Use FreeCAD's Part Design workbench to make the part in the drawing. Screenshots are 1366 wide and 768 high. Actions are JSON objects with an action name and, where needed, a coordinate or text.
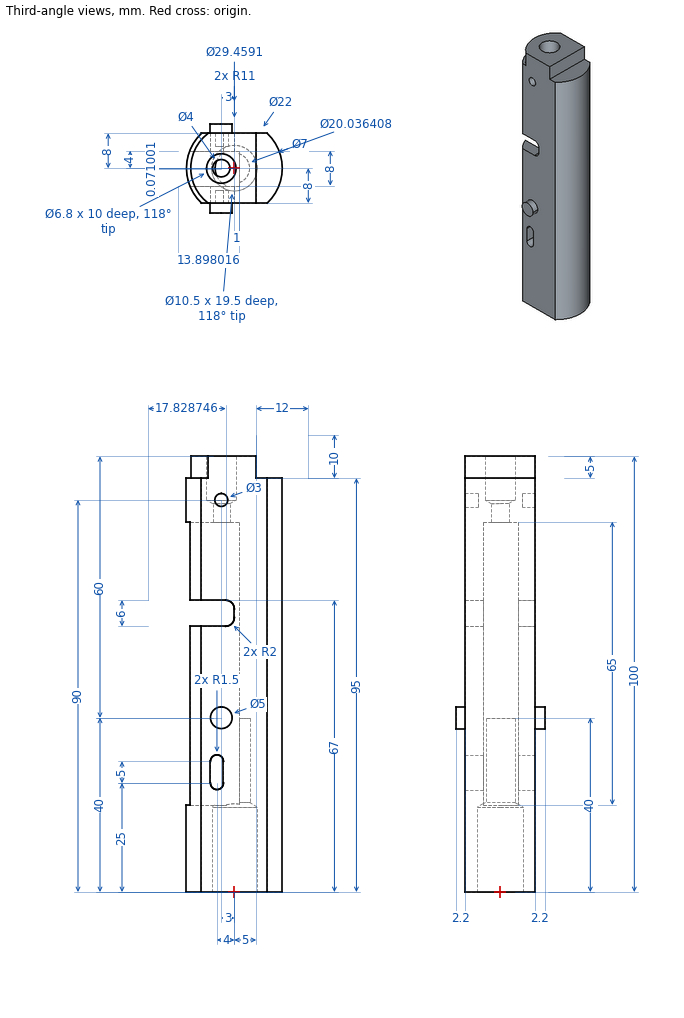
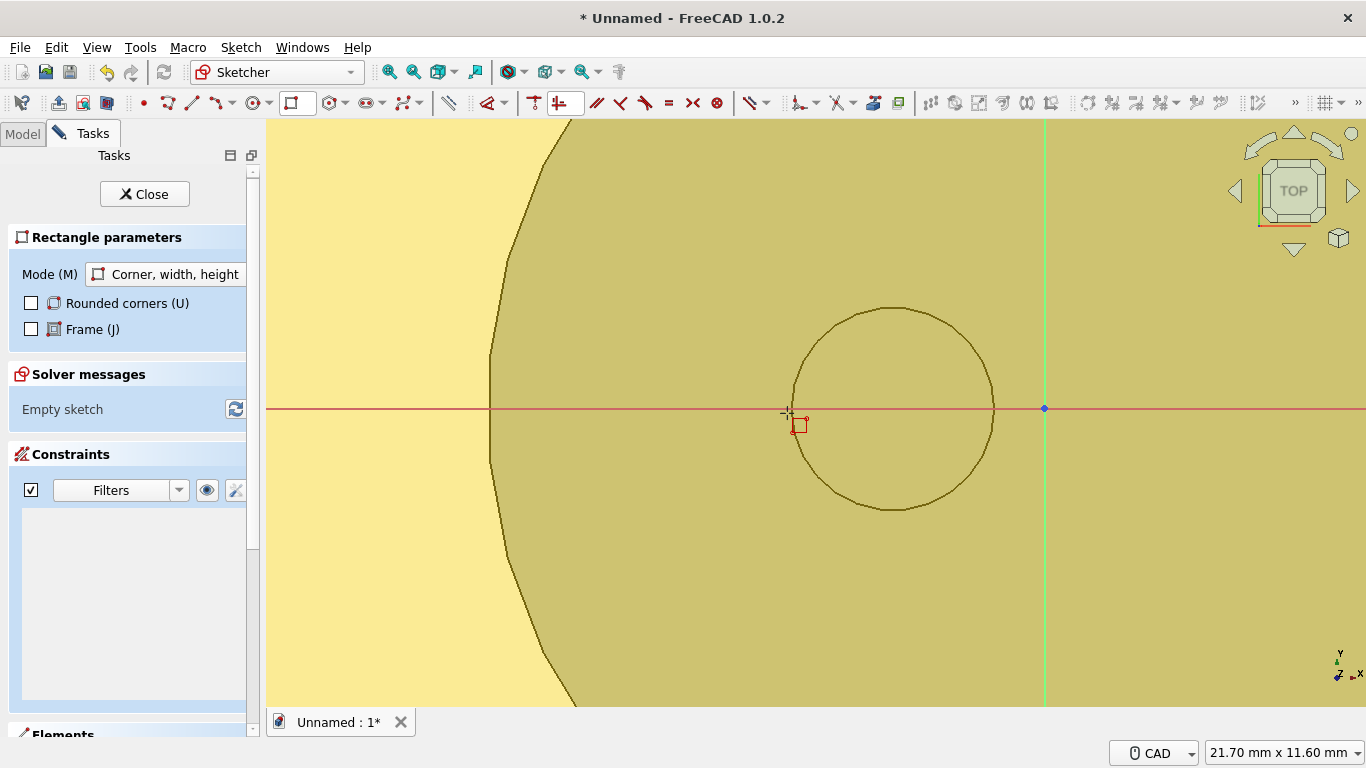
{"action": "left_click", "coordinate": [391, 206]}
{"action": "mouse_move", "coordinate": [1096, 612]}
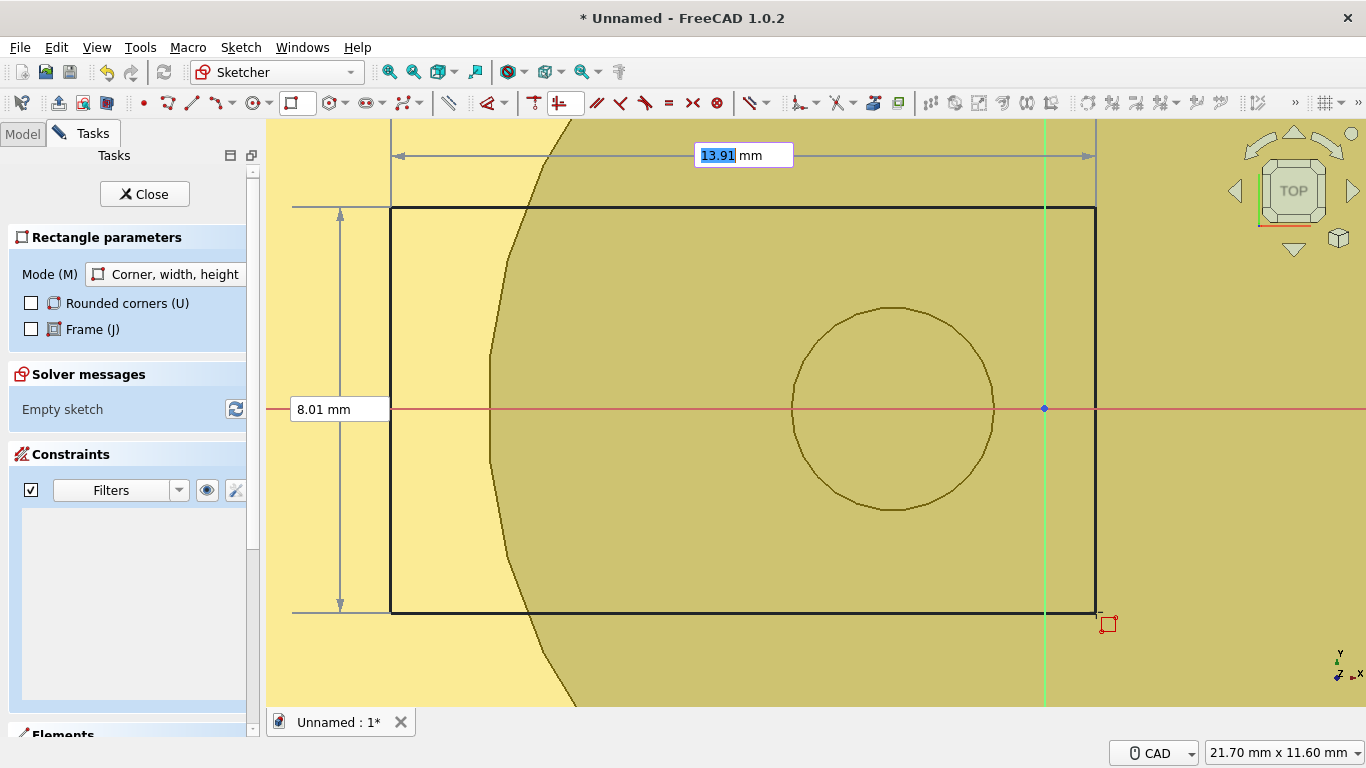
{"action": "type", "text": "13.898016"}
{"action": "key", "text": "Tab"}
{"action": "type", "text": "8"}
{"action": "key", "text": "Return"}
{"action": "key", "text": "Escape"}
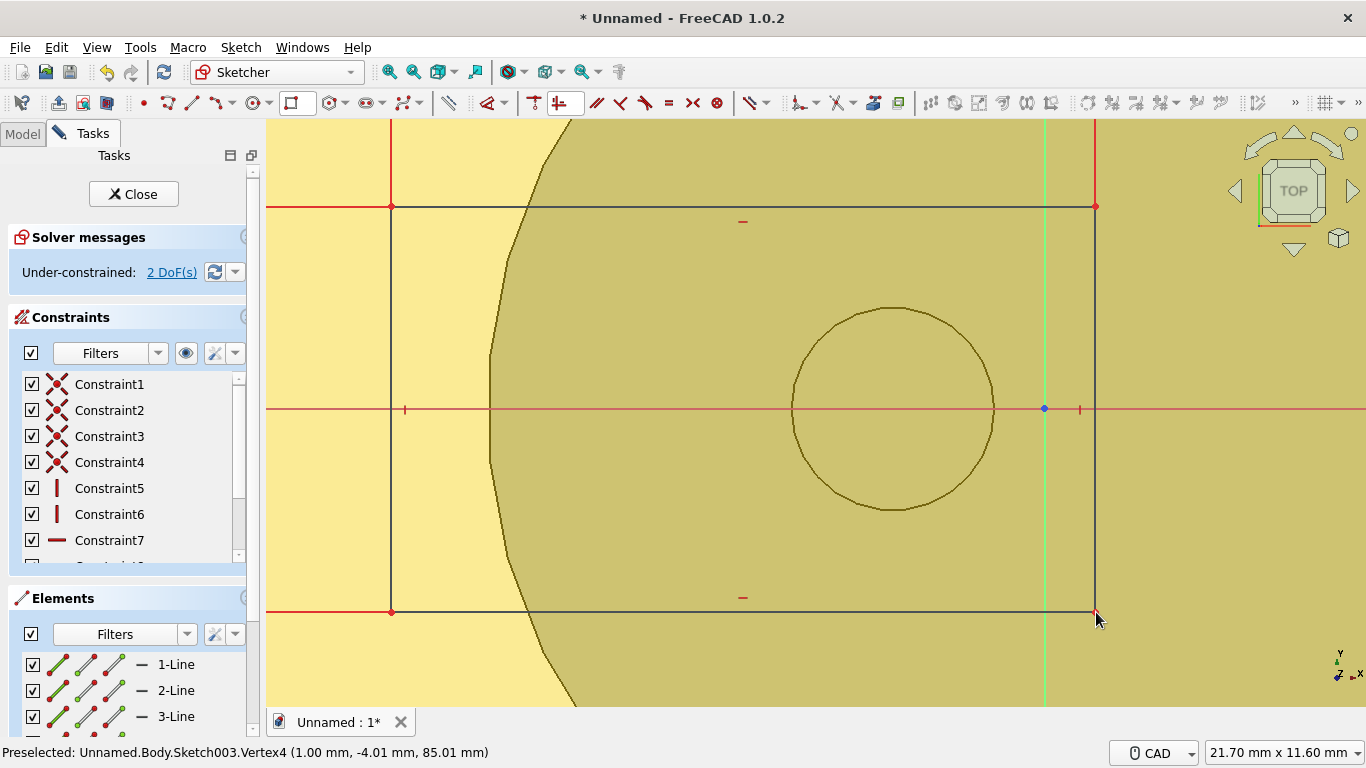
{"action": "key", "text": "d"}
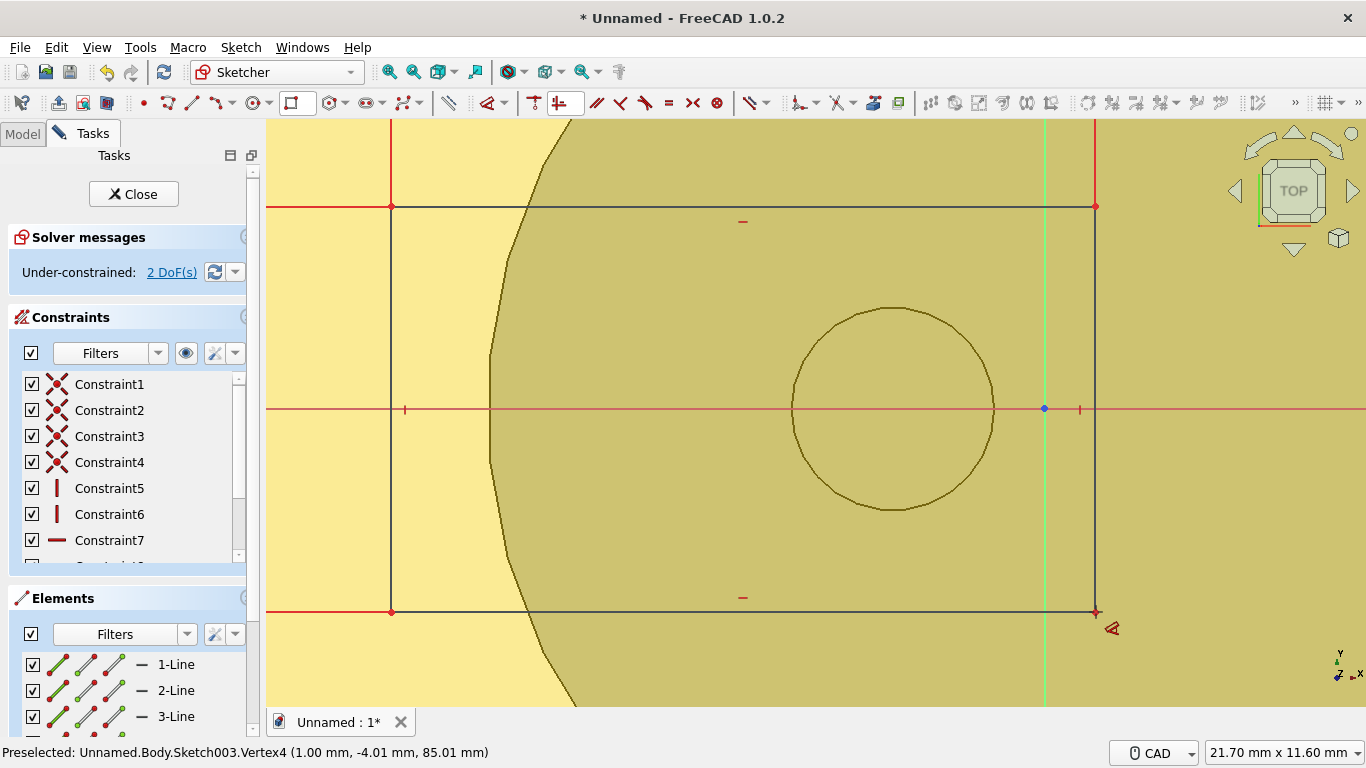
{"action": "left_click", "coordinate": [391, 207]}
{"action": "left_click", "coordinate": [357, 308]}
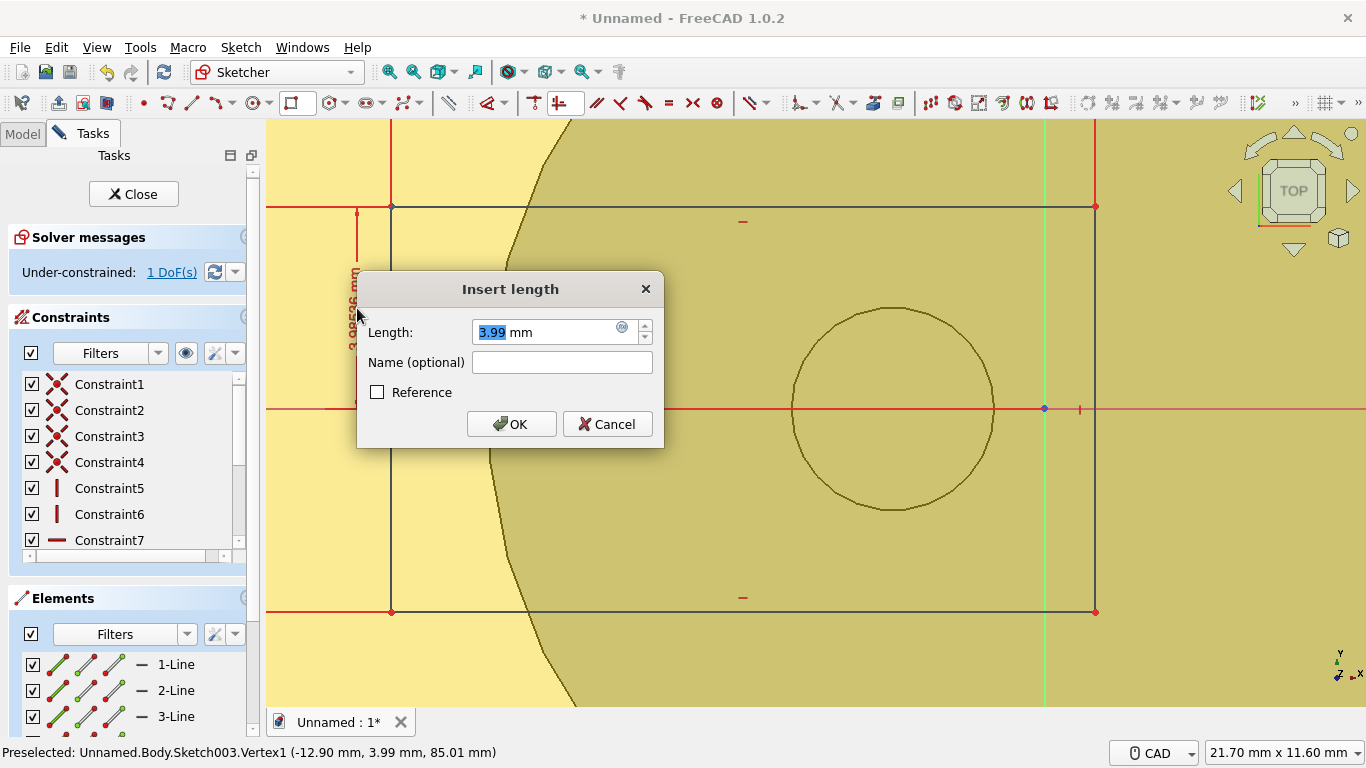
{"action": "type", "text": "4"}
{"action": "key", "text": "Return"}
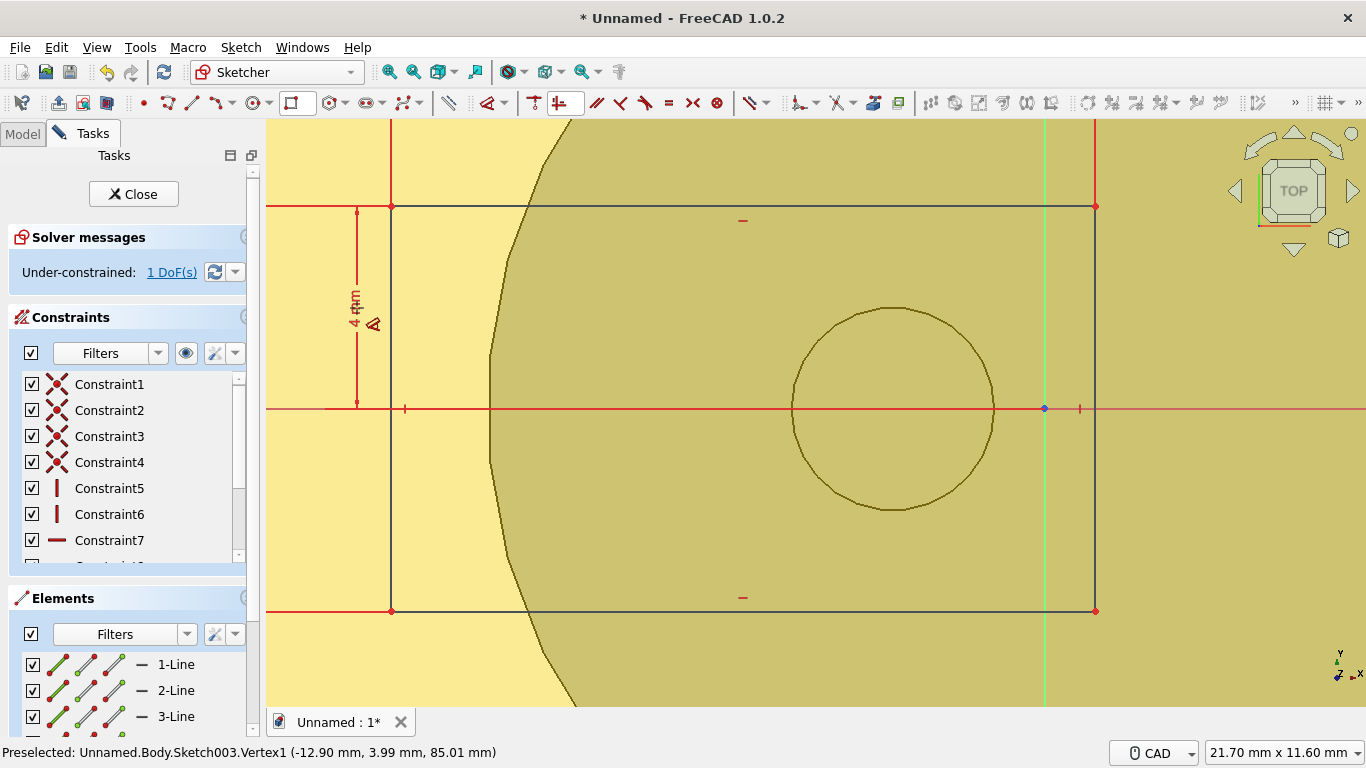
{"action": "left_click", "coordinate": [1095, 612]}
{"action": "left_click", "coordinate": [1070, 646]}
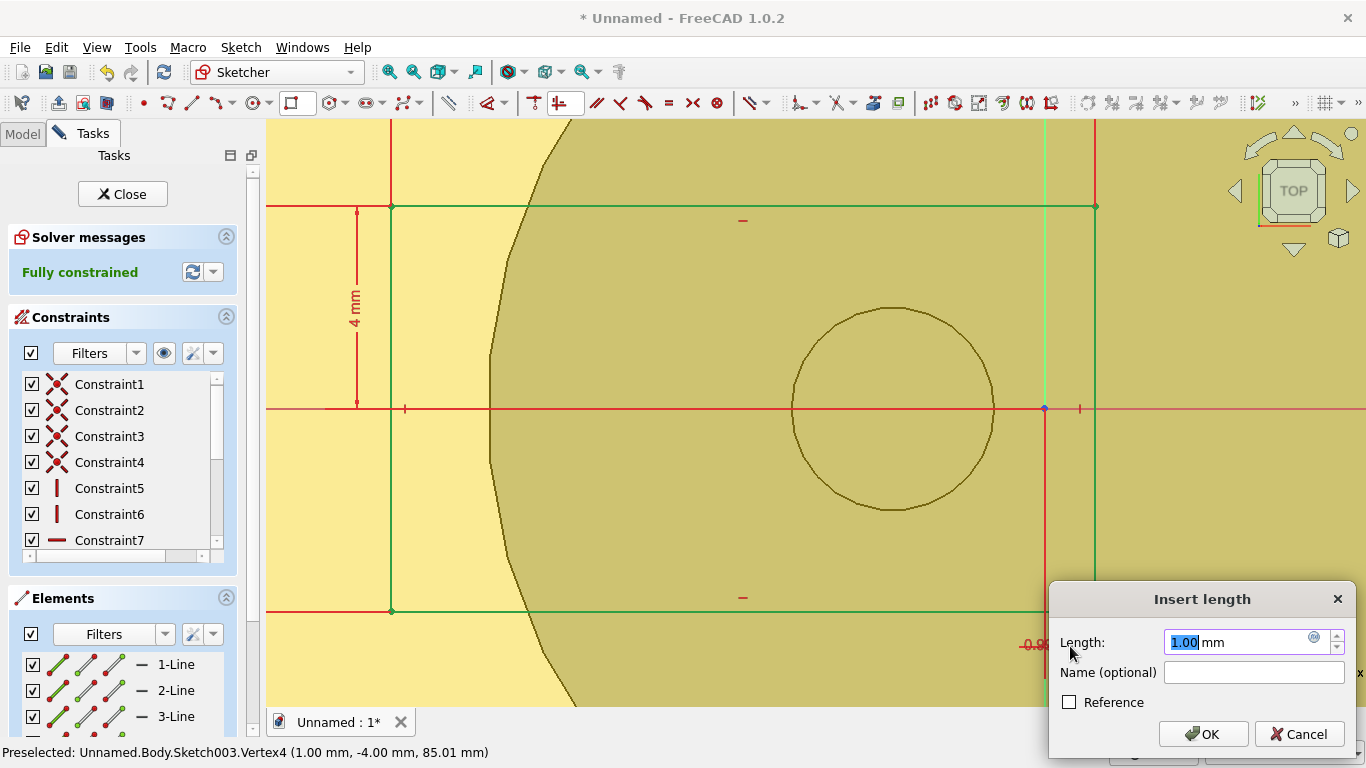
{"action": "type", "text": "1"}
{"action": "key", "text": "Return"}
{"action": "key", "text": "Escape"}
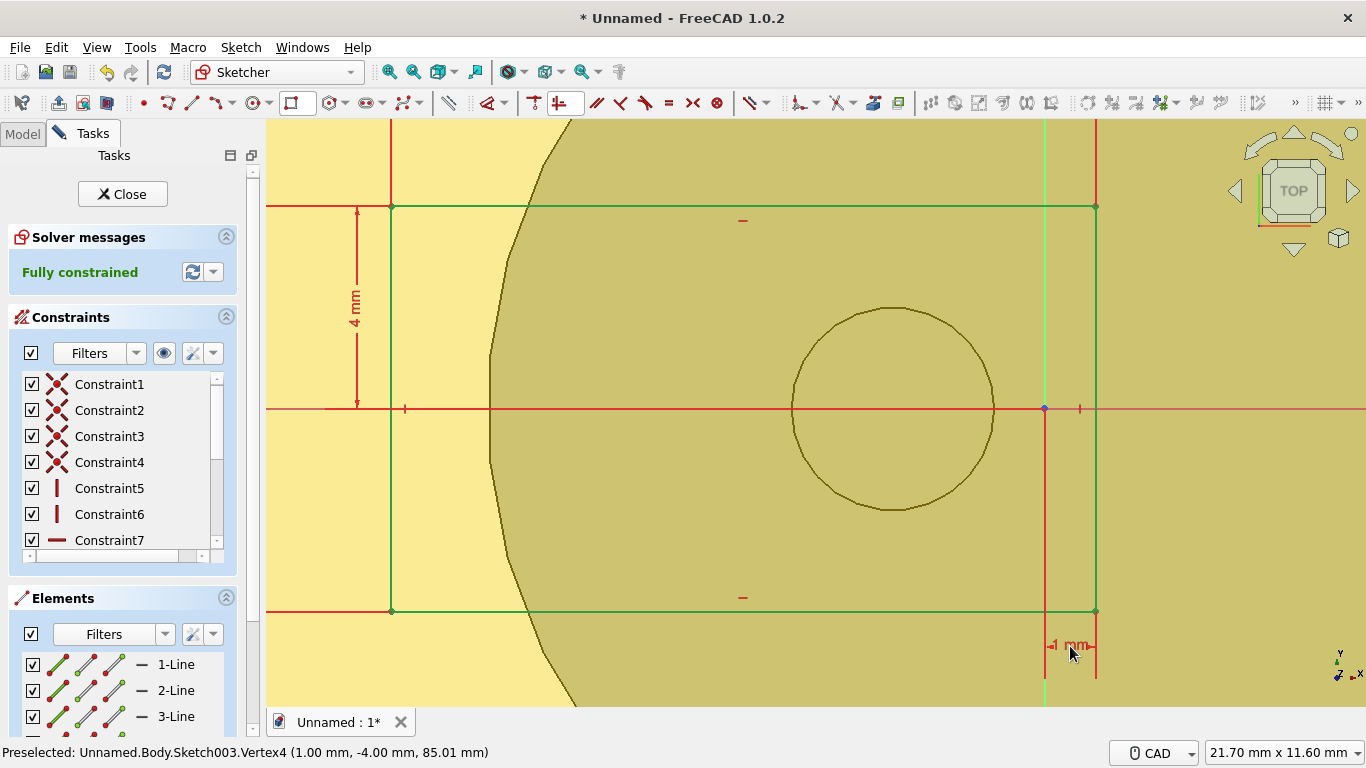
{"action": "left_click", "coordinate": [123, 194]}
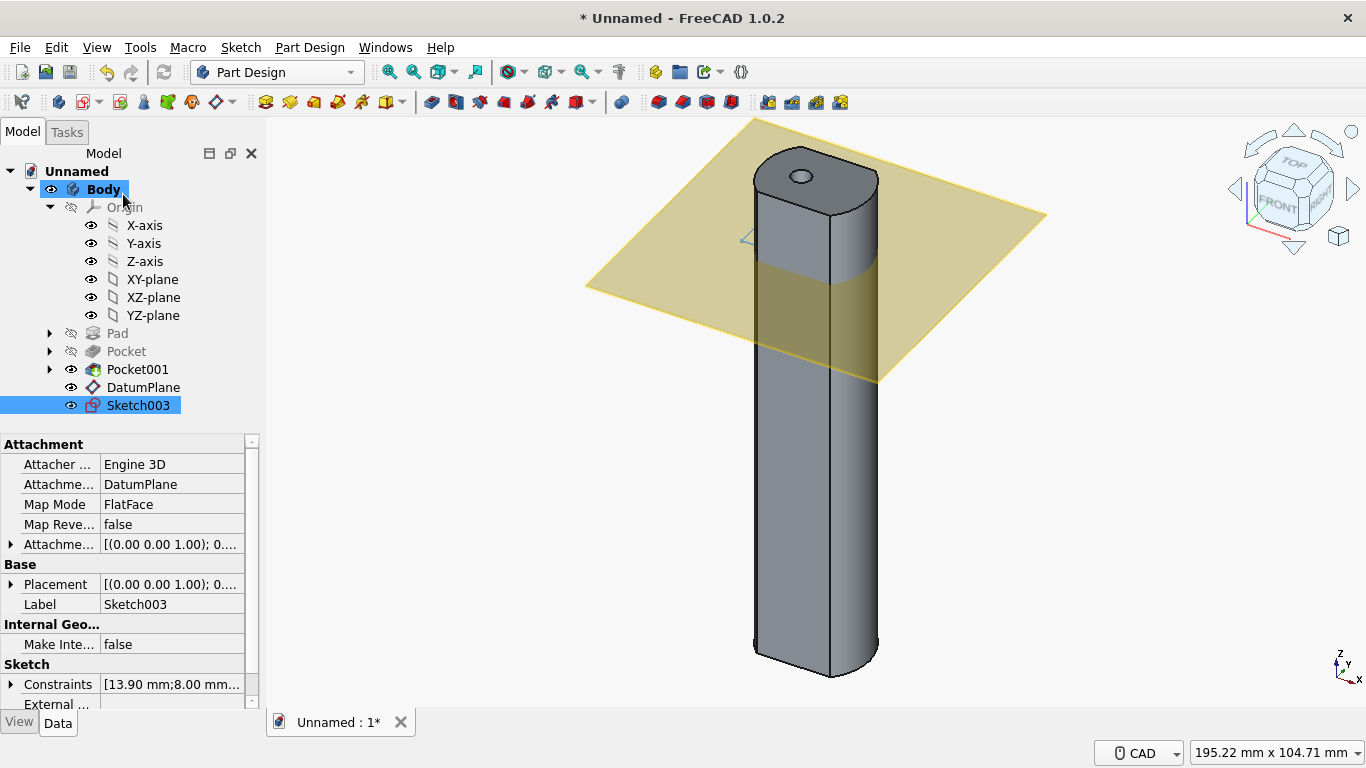
{"action": "left_click", "coordinate": [432, 102]}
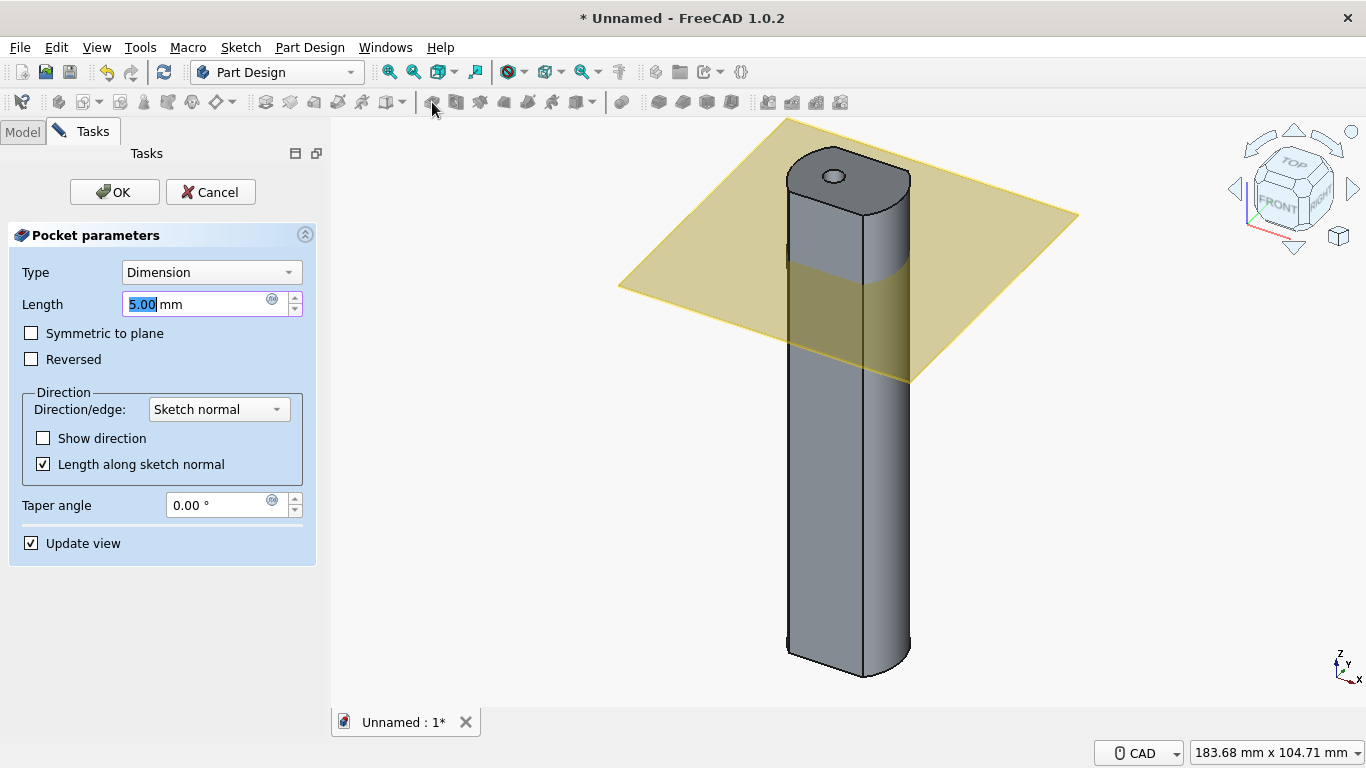
{"action": "type", "text": "65"}
{"action": "key", "text": "Tab"}